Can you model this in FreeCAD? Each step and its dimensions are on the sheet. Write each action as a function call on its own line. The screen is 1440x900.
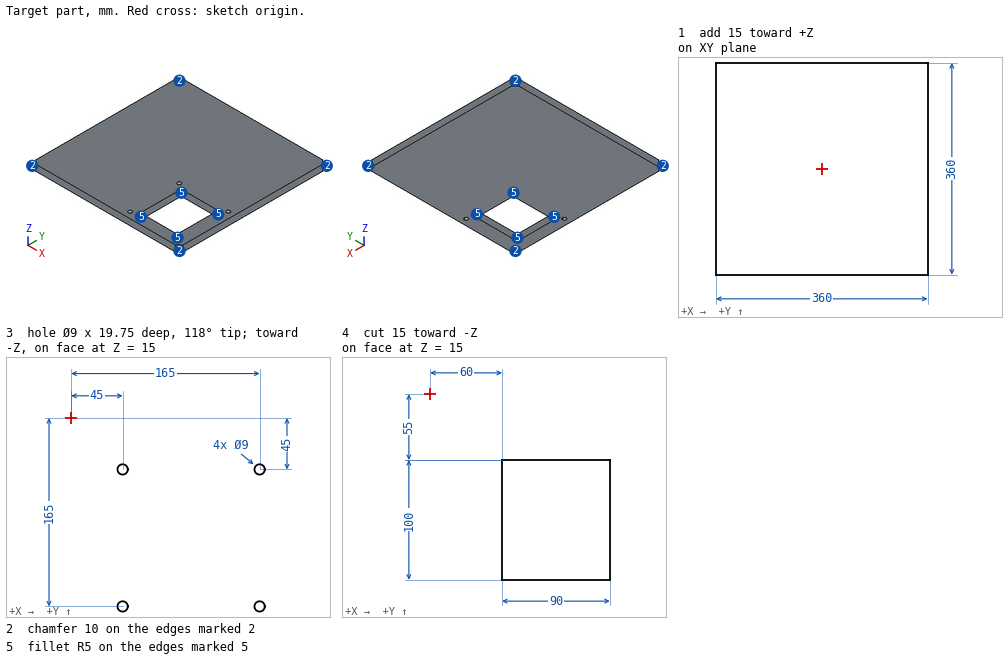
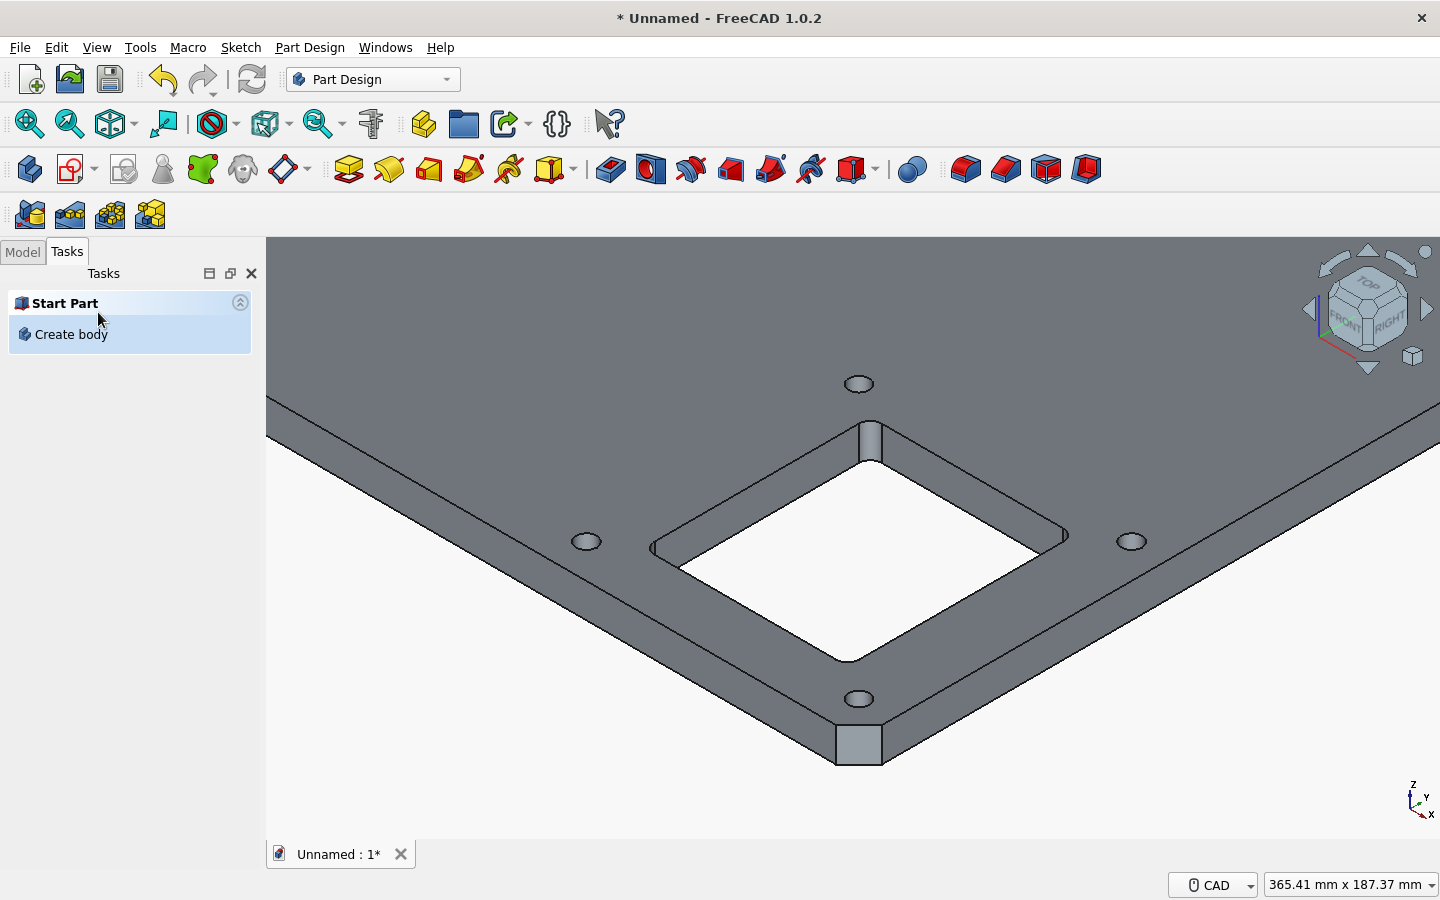
key(v)
key(f)